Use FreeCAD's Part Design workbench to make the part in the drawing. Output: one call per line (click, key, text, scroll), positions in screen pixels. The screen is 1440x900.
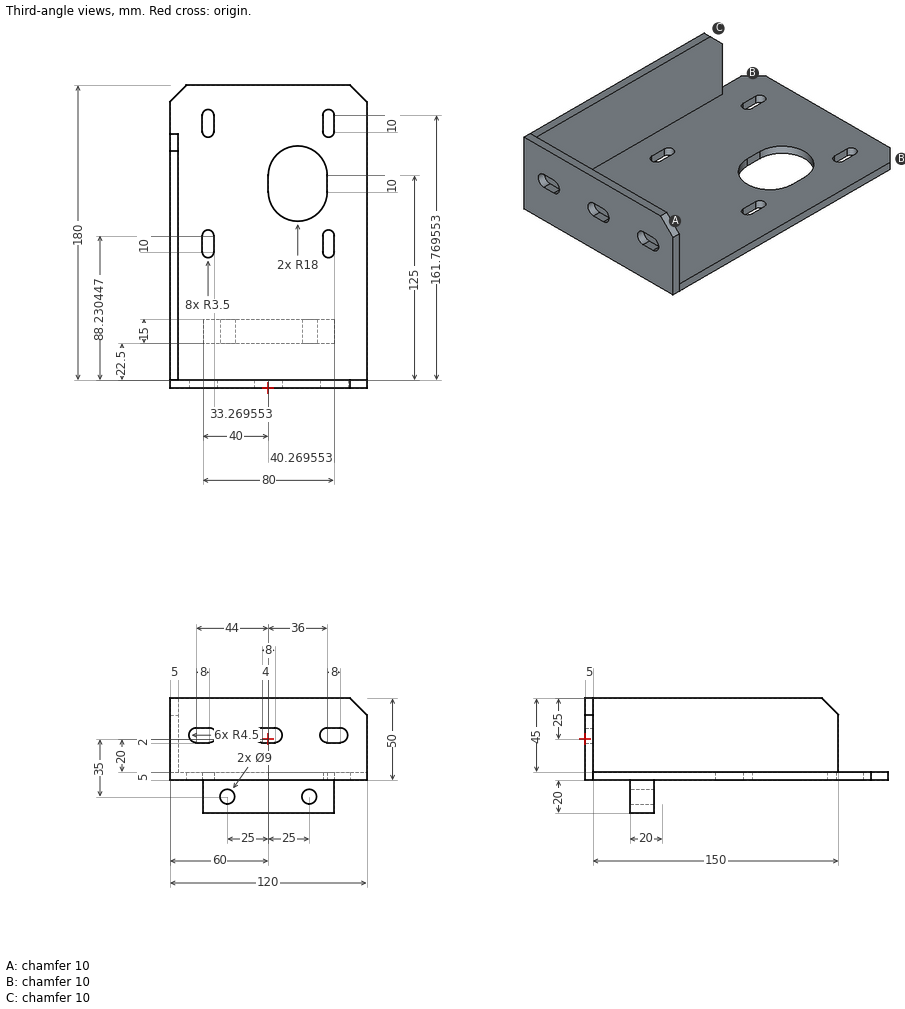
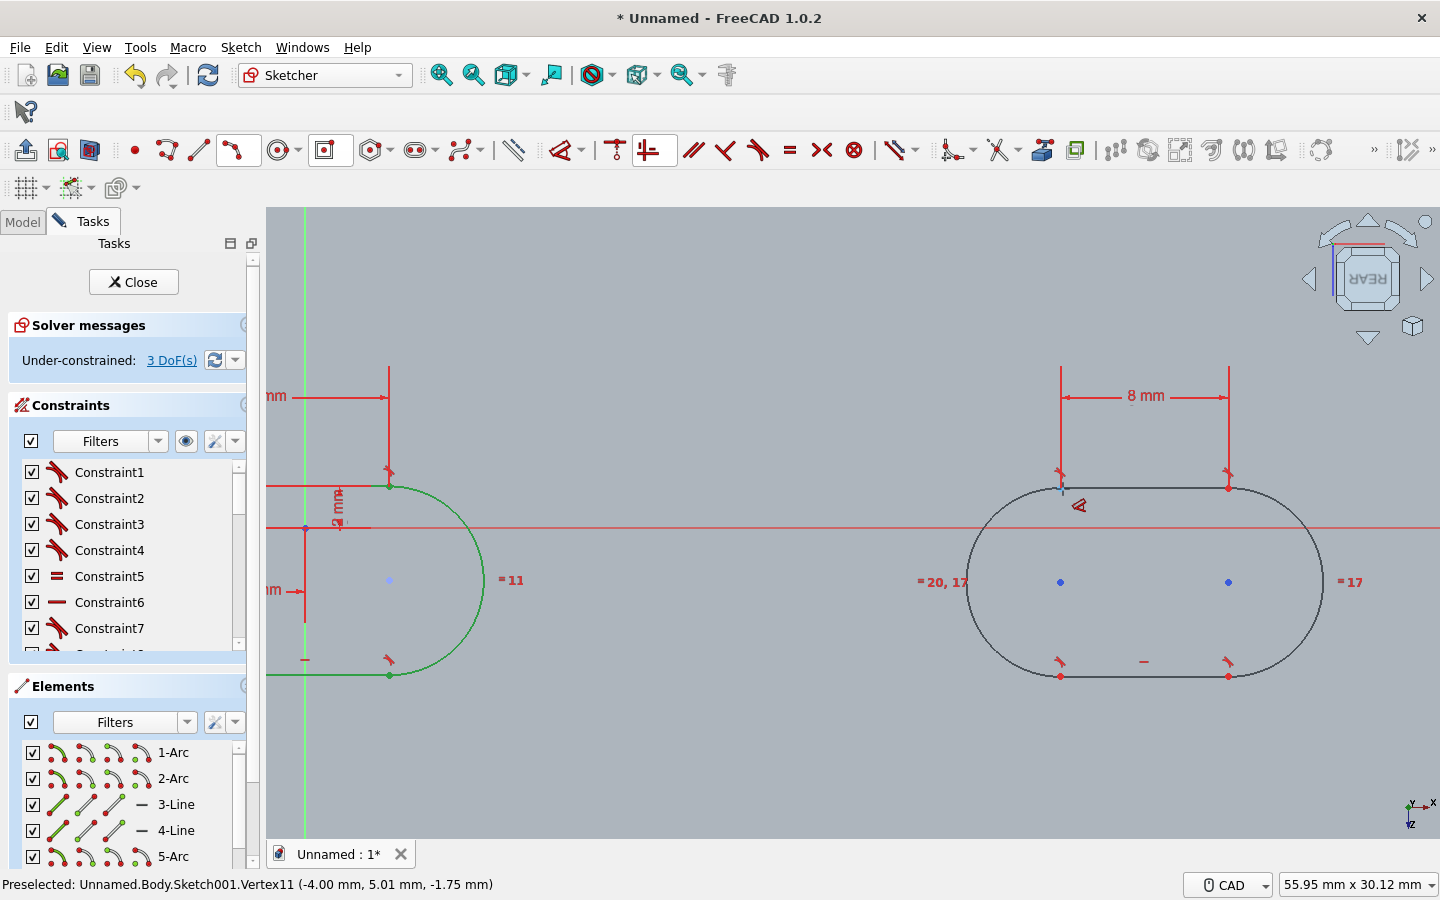
click(1061, 488)
click(1095, 508)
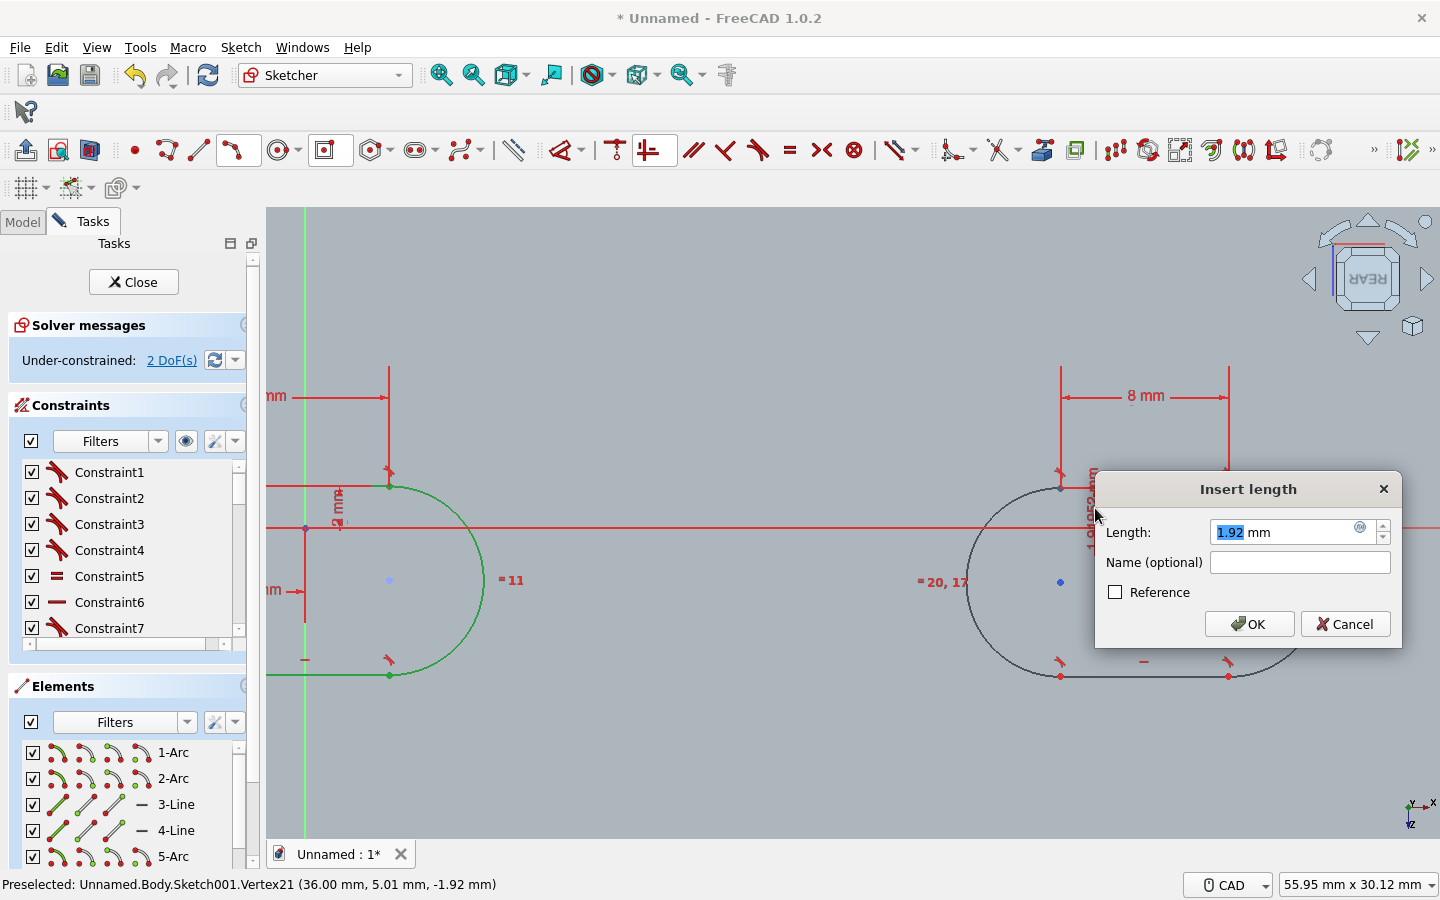
text(2)
key(Return)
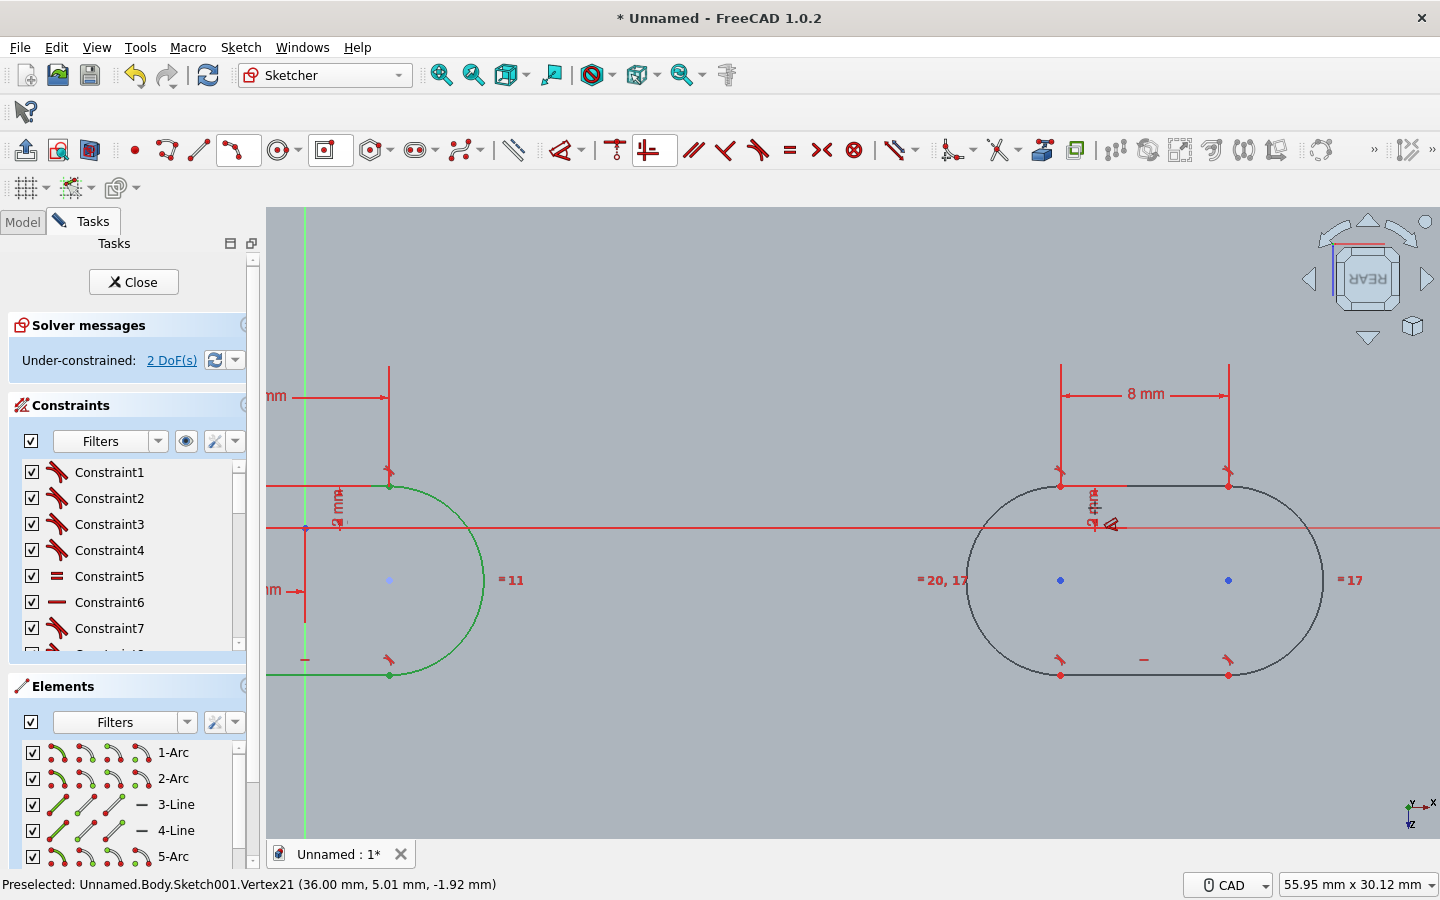
scroll(1063, 489, down, 5)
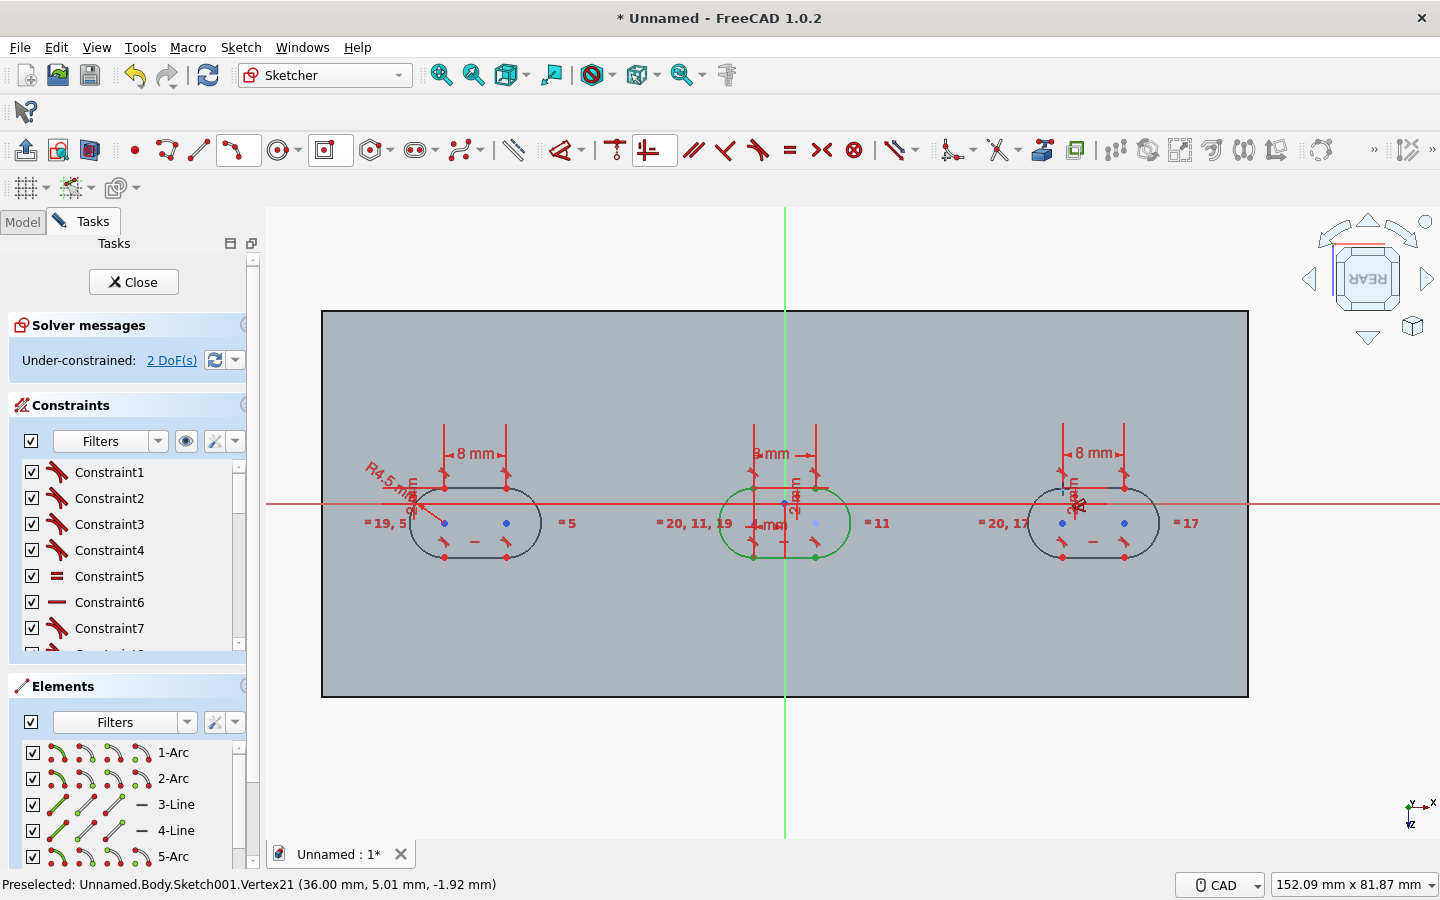
click(445, 488)
click(615, 454)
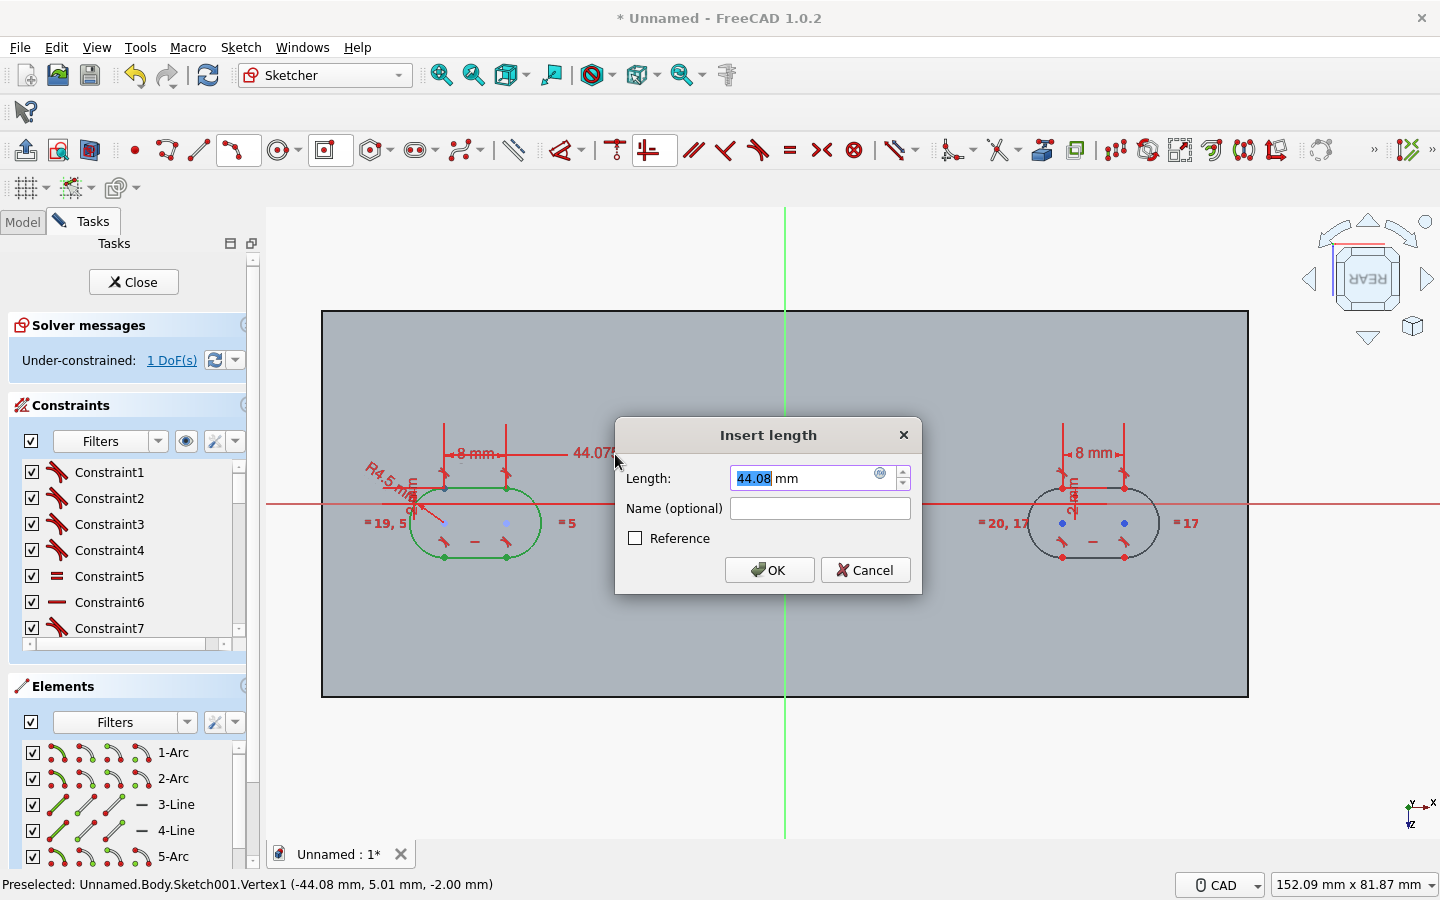
text(44)
key(Return)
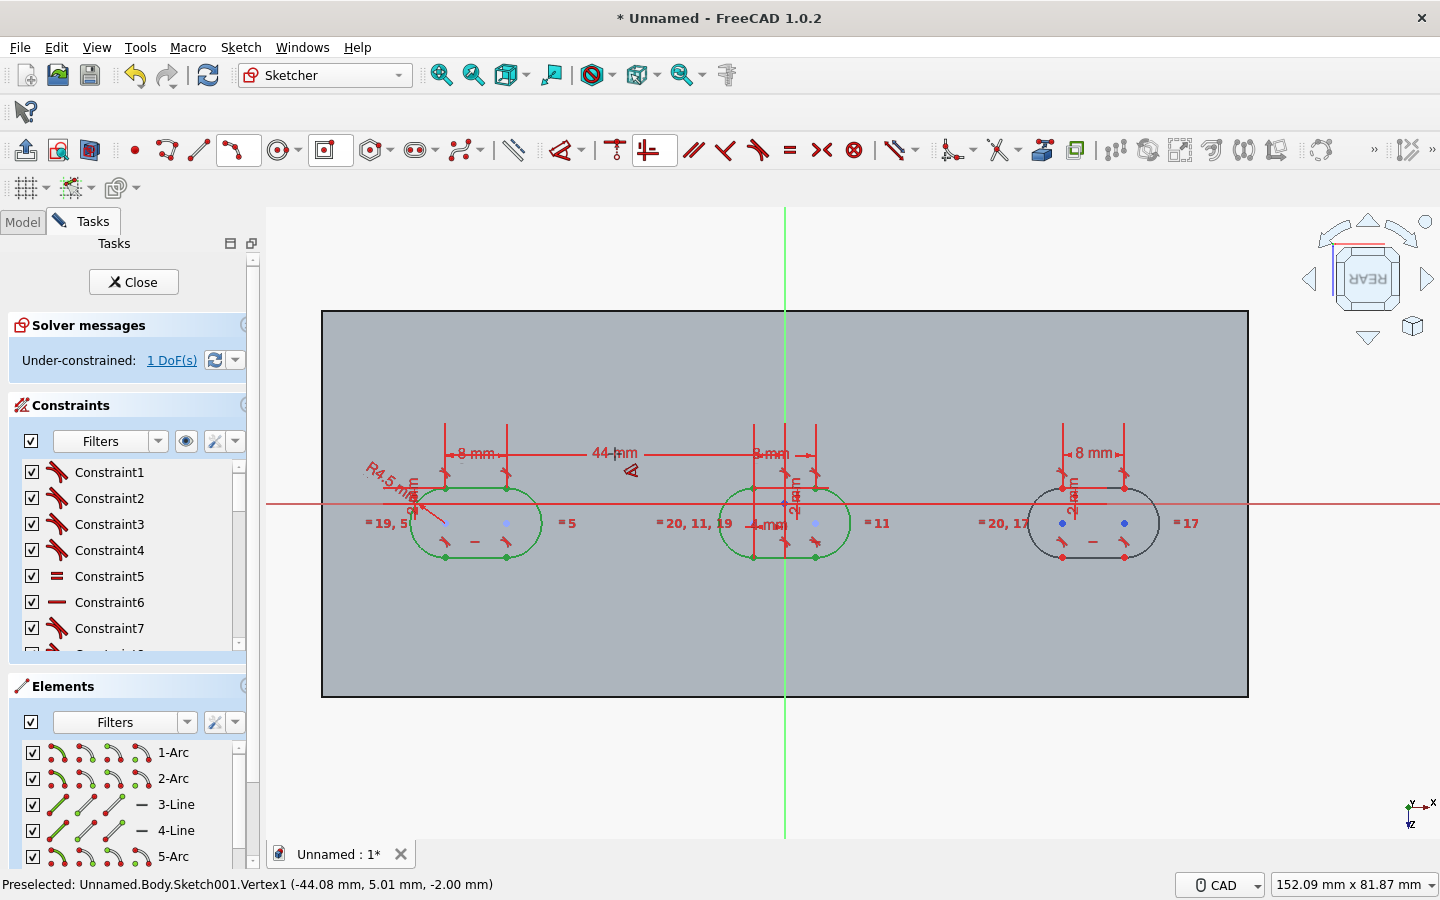
click(1063, 488)
click(924, 454)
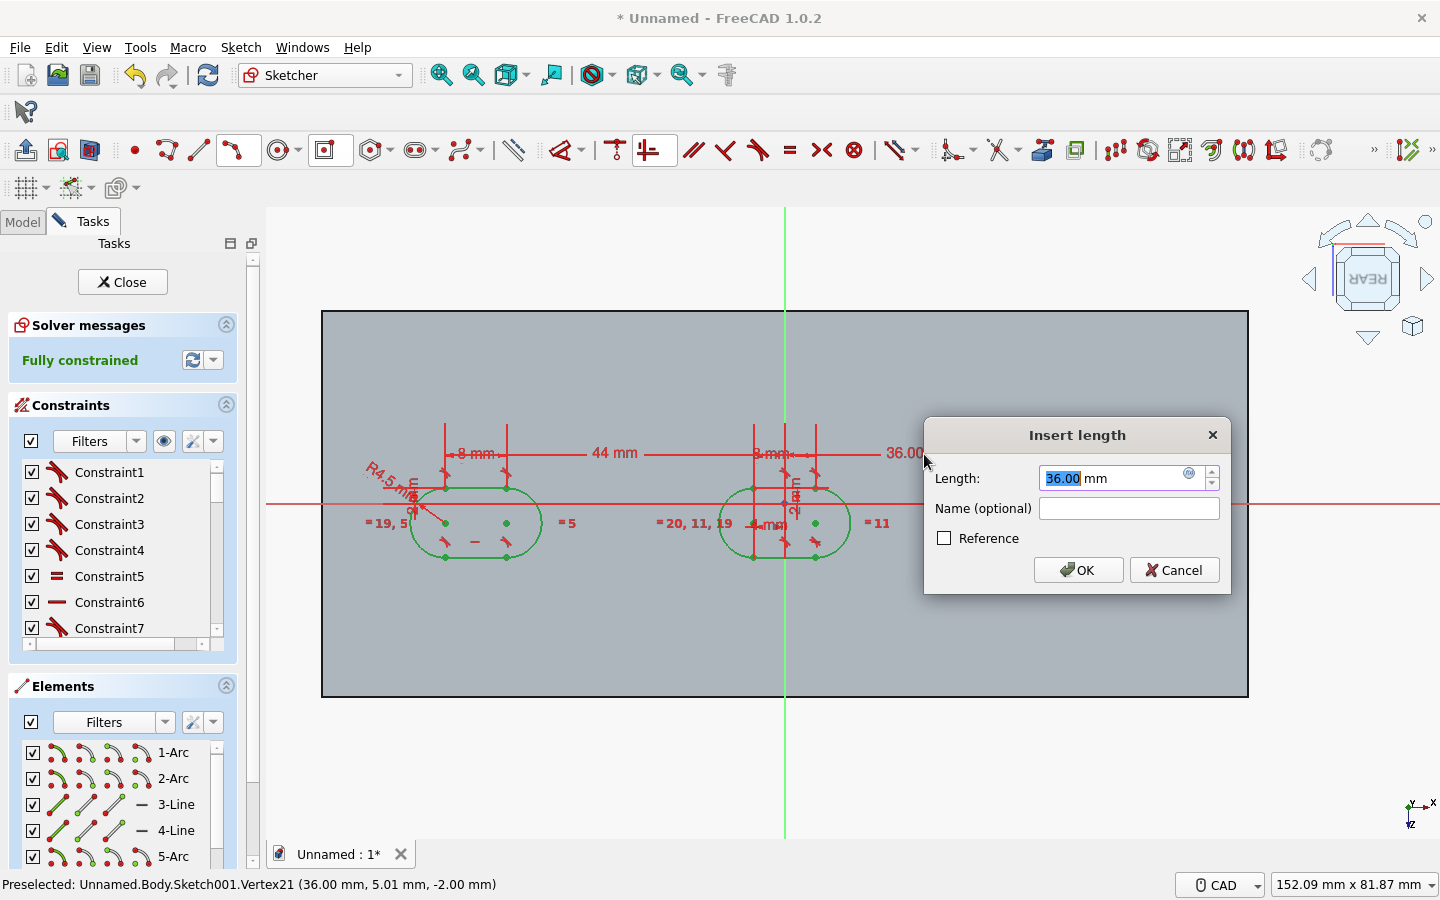
text(36)
key(Return)
key(Escape)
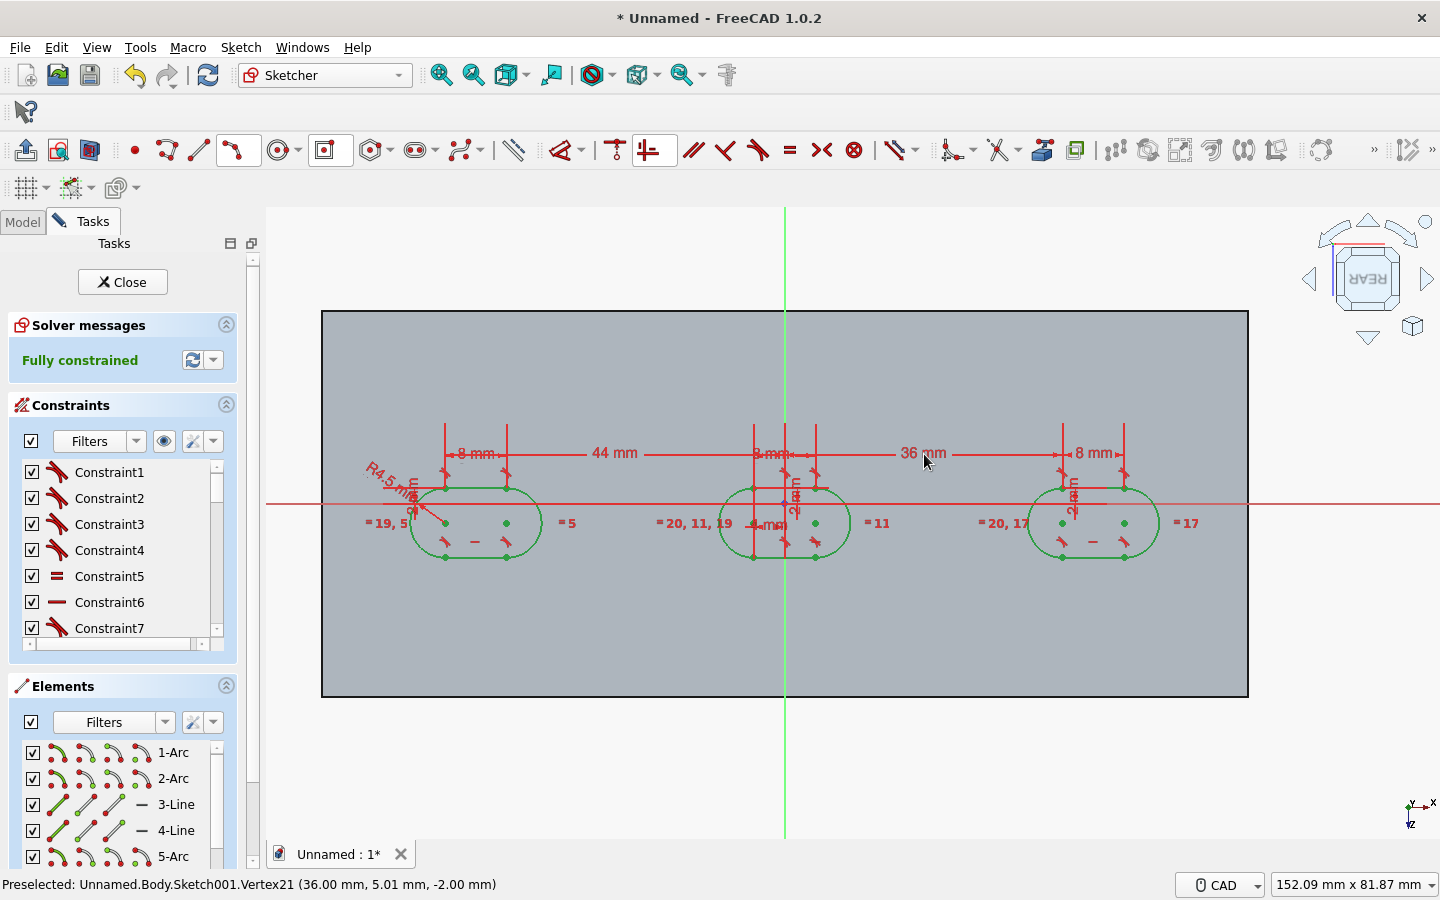
click(123, 282)